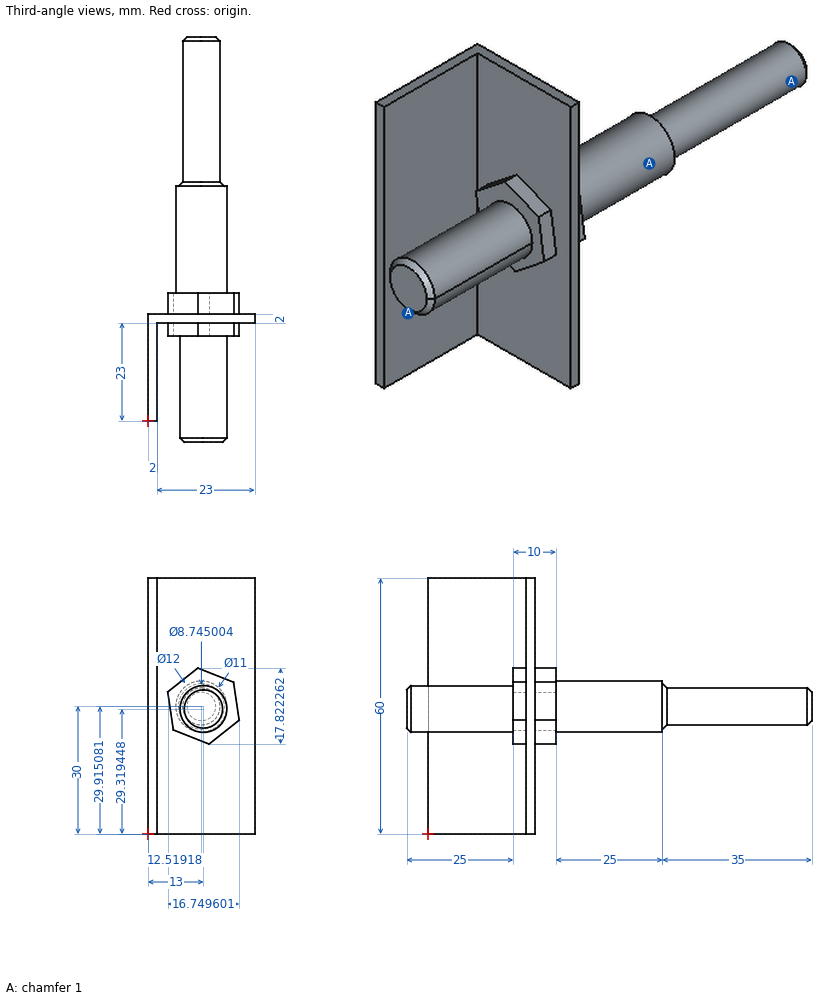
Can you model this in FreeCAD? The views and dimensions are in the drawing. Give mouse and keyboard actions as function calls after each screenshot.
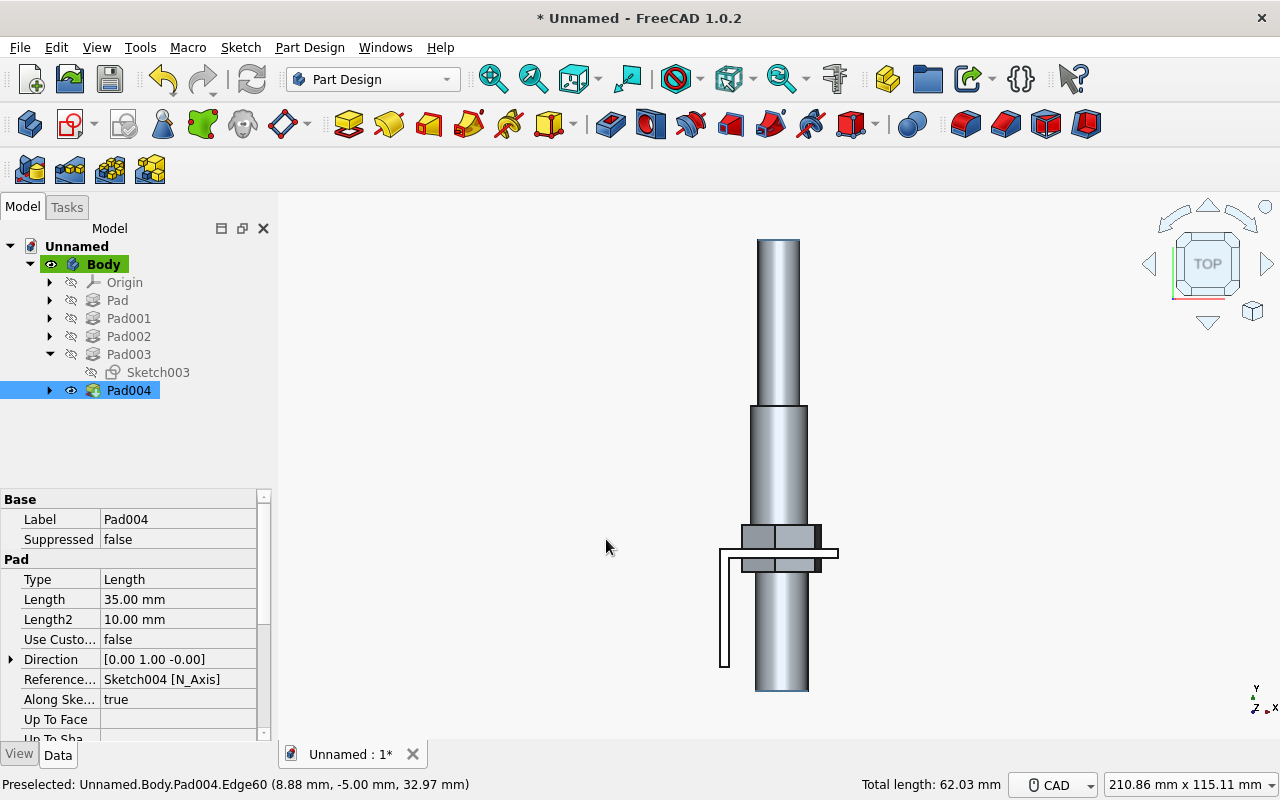
key(1)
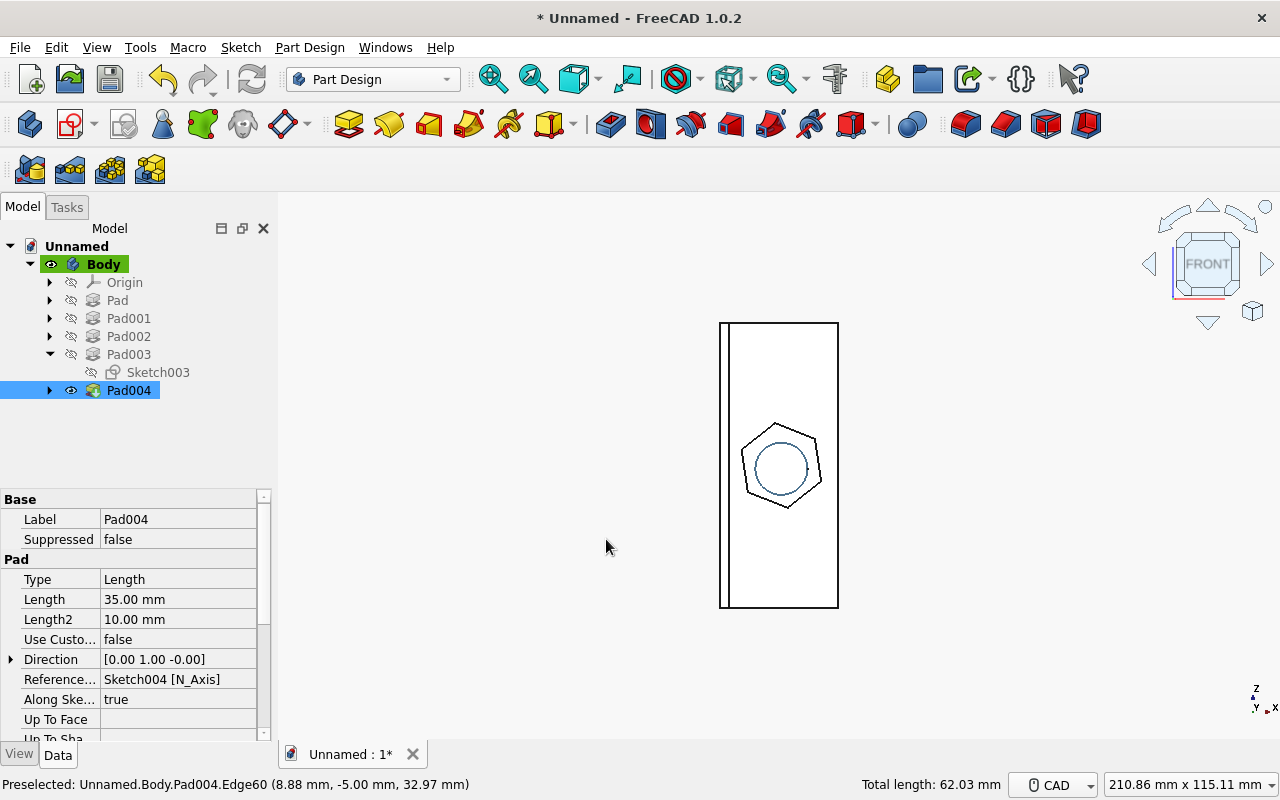
key(3)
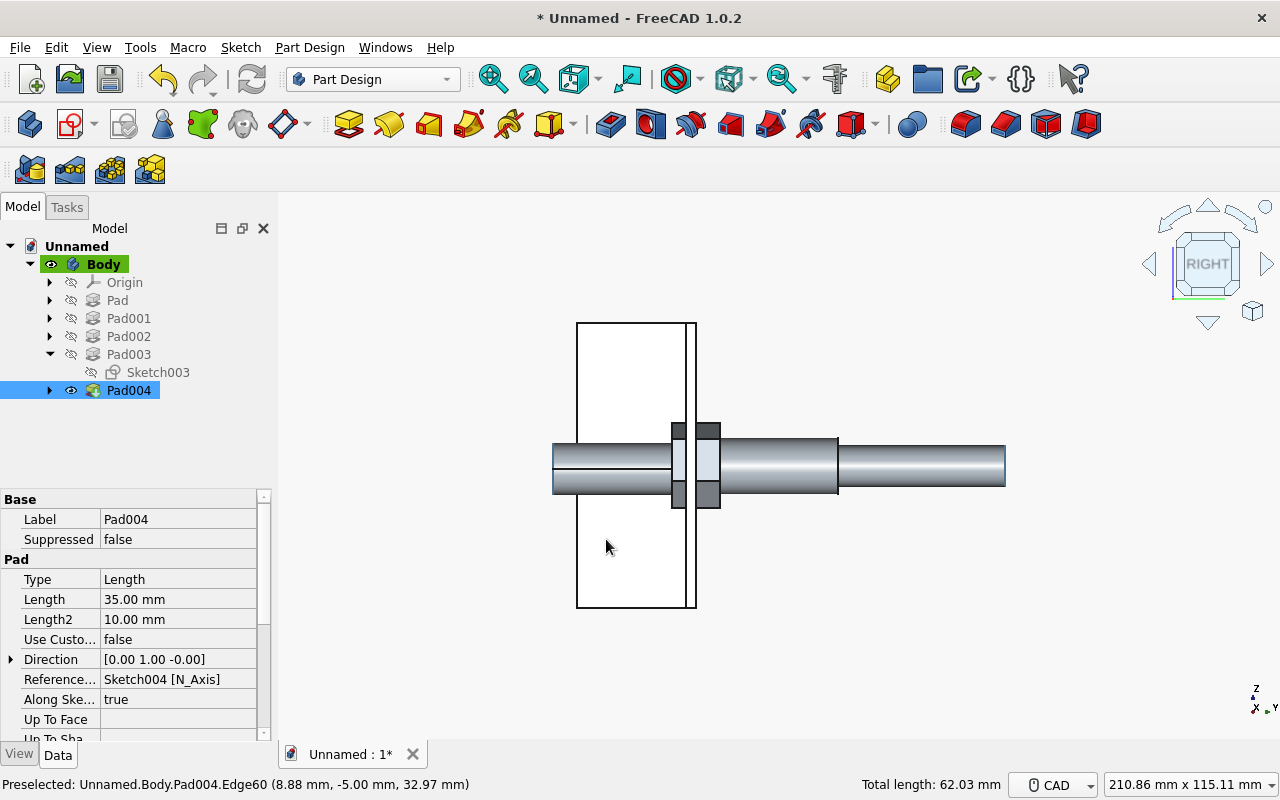
key(5)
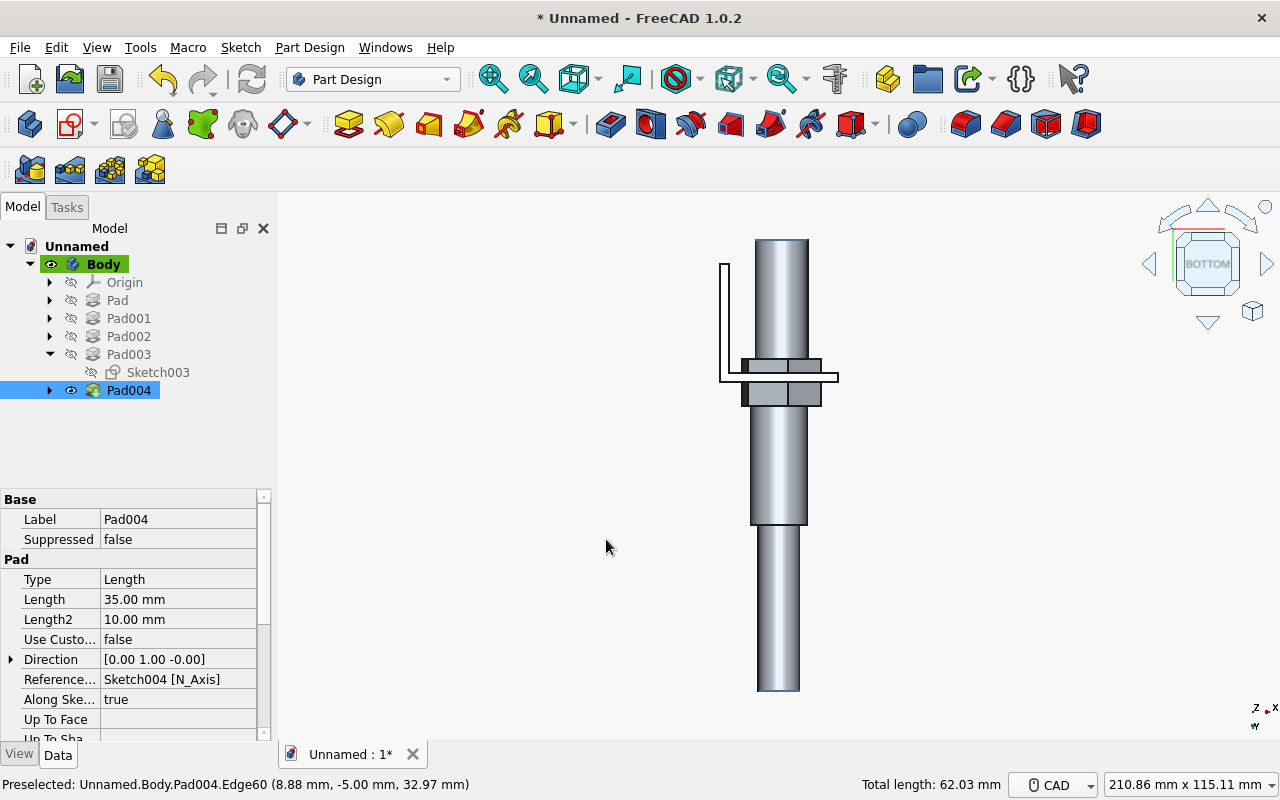
key(4)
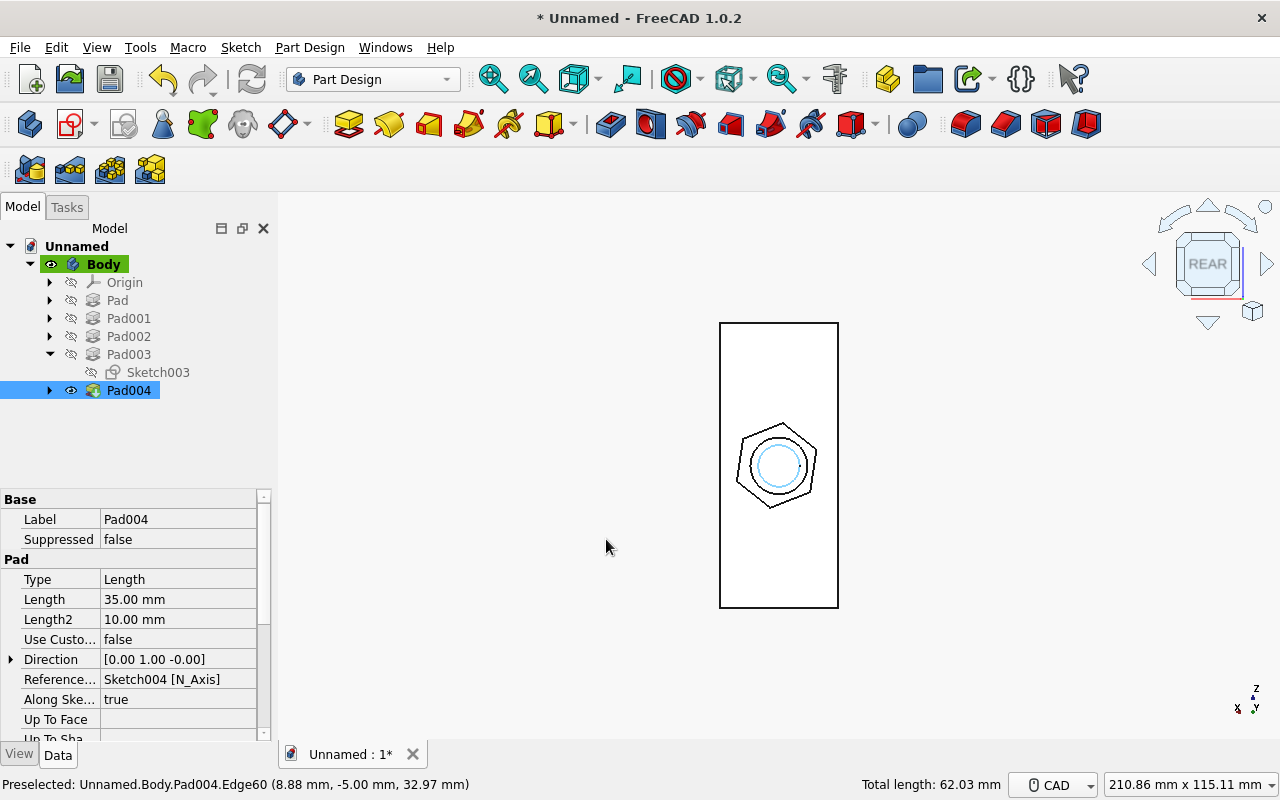
key(6)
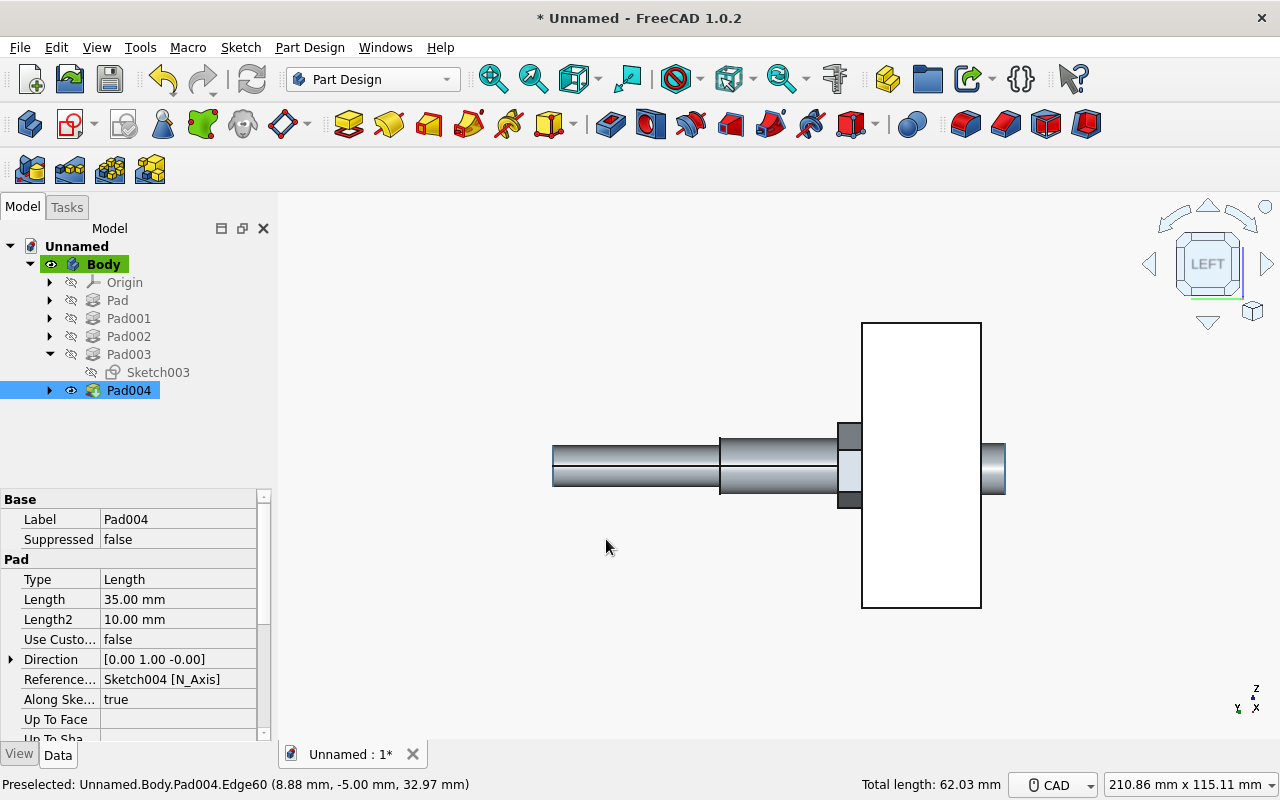
key(v)
key(3)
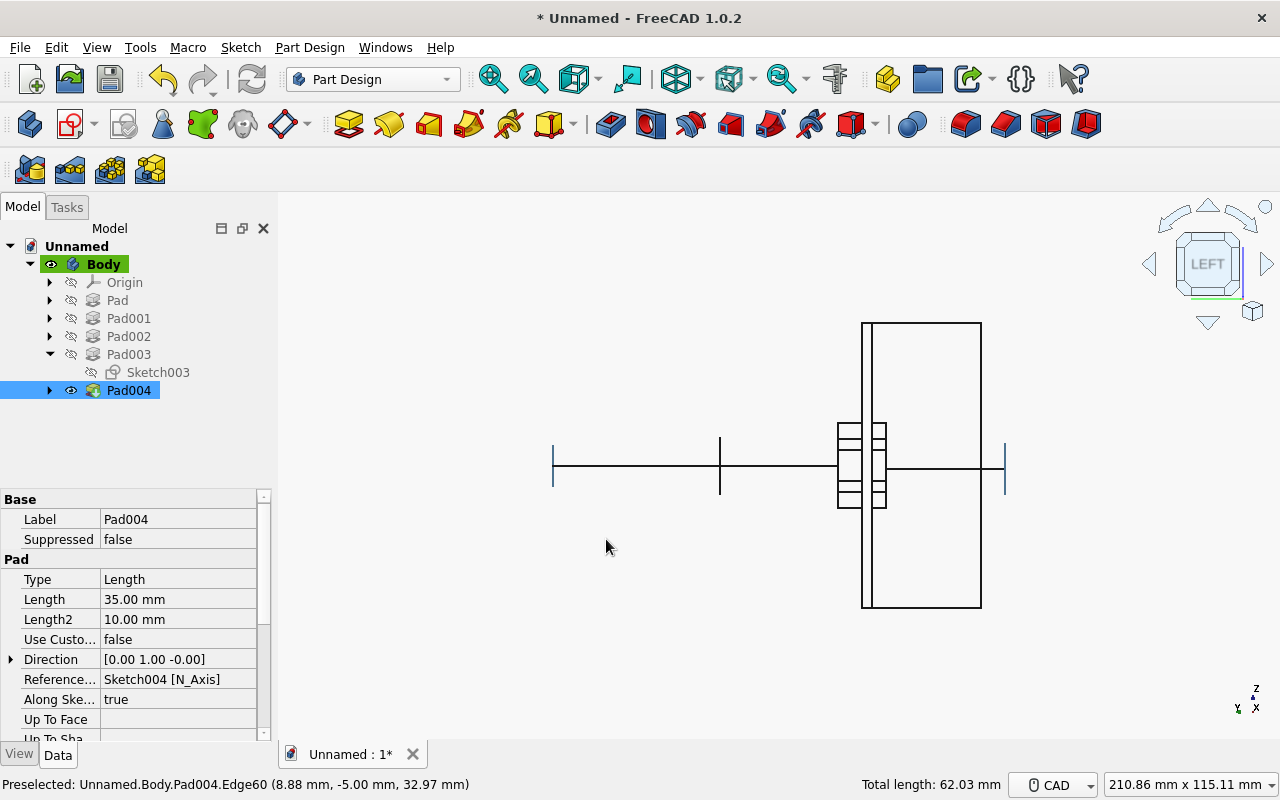
key(0)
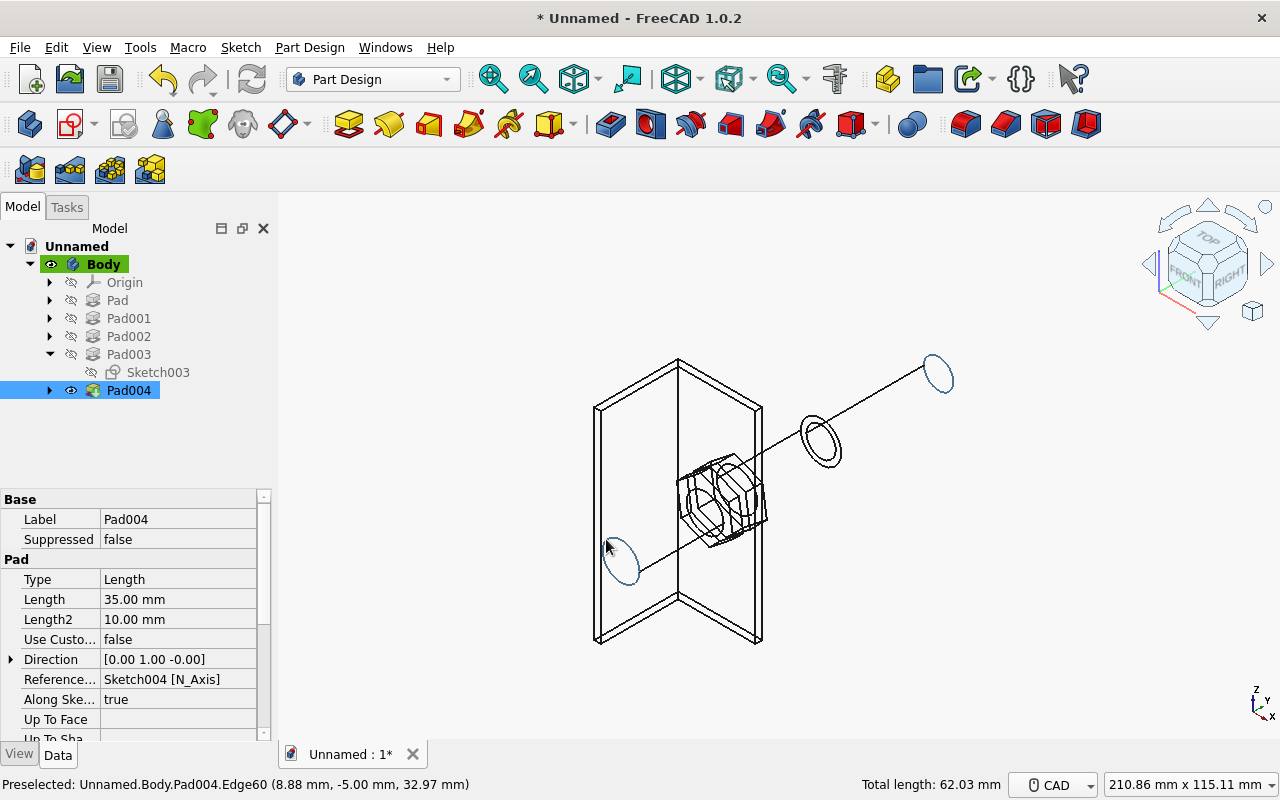
click(833, 457, ctrl)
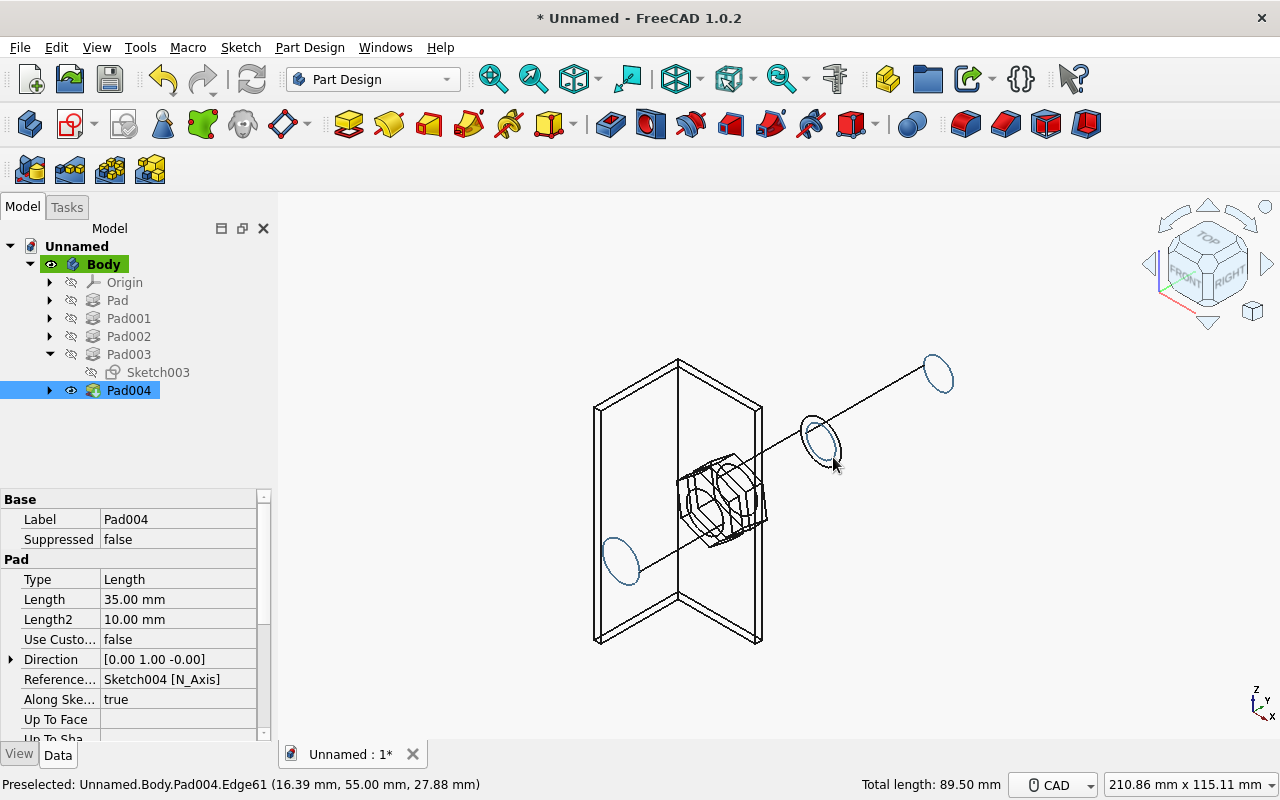
key(v)
key(1)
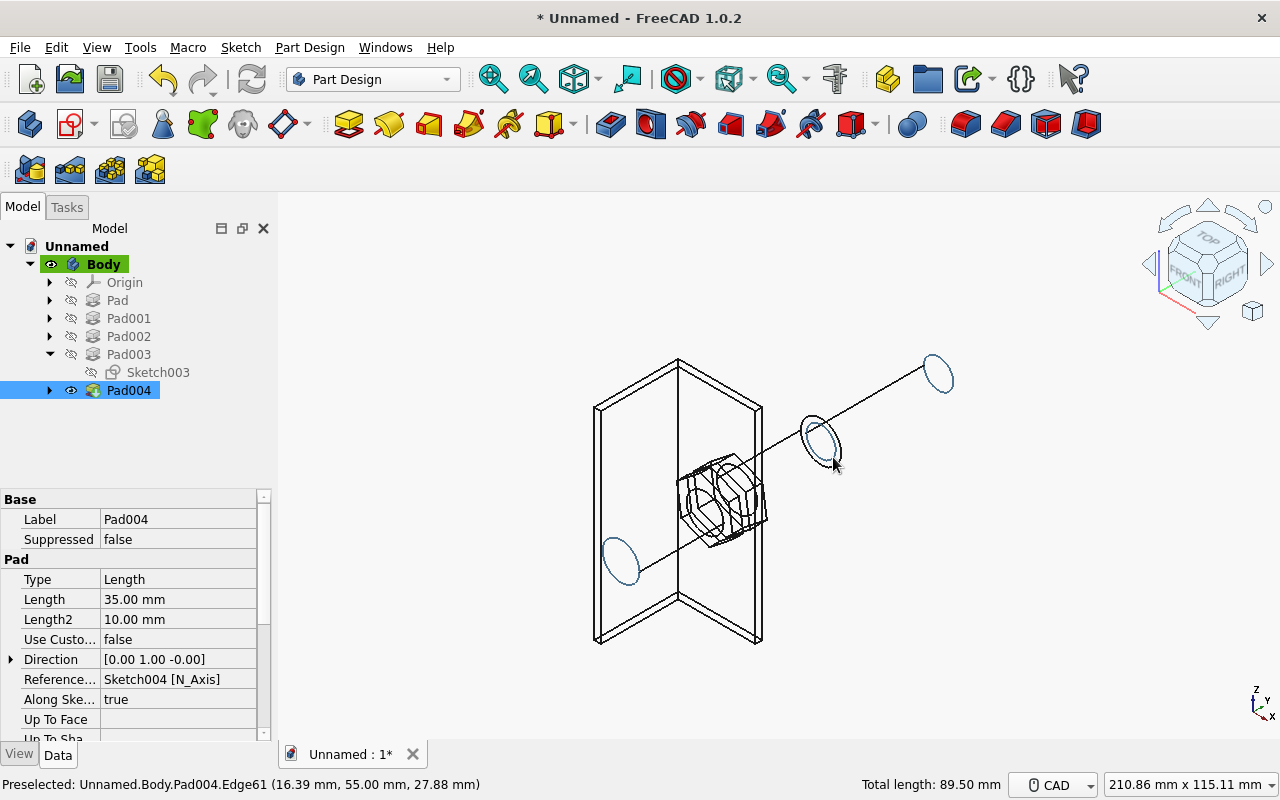
click(1006, 124)